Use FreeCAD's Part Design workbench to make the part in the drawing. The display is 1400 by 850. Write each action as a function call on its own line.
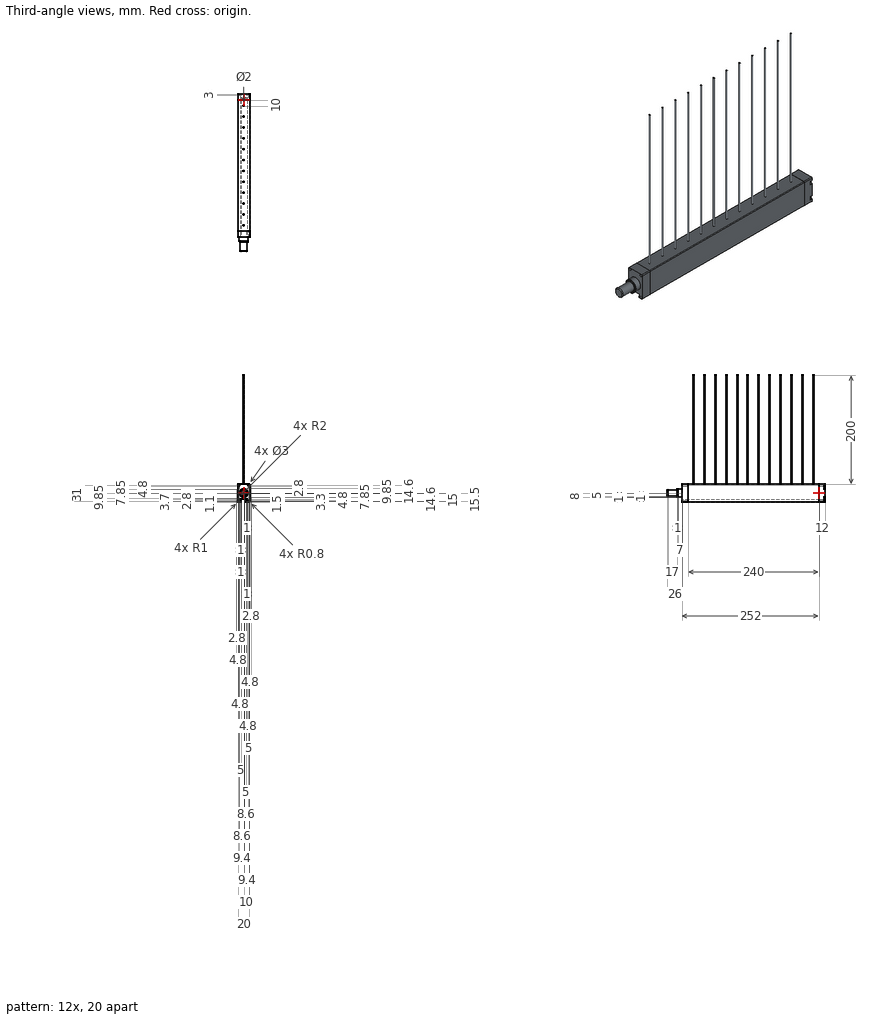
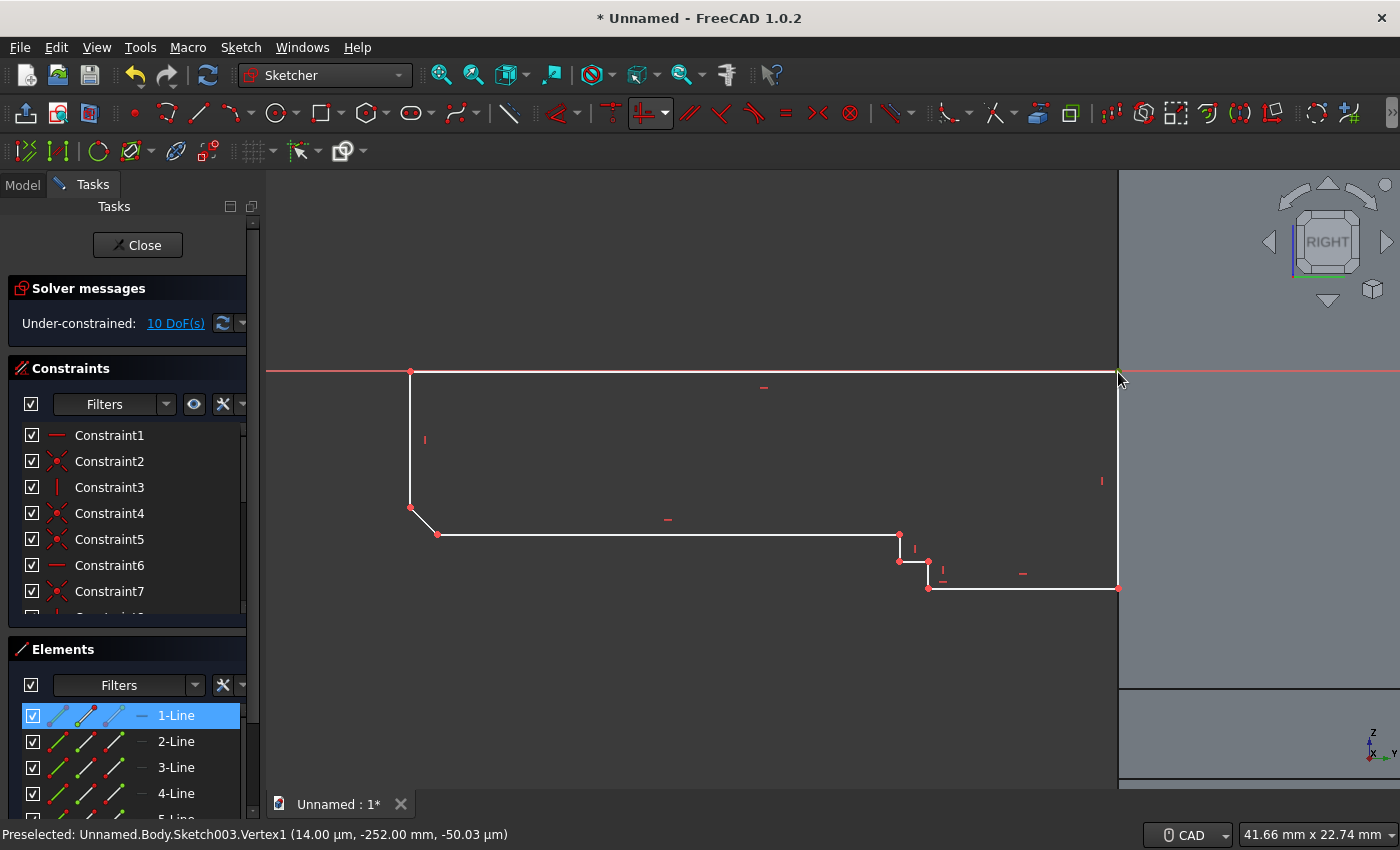
click(361, 371)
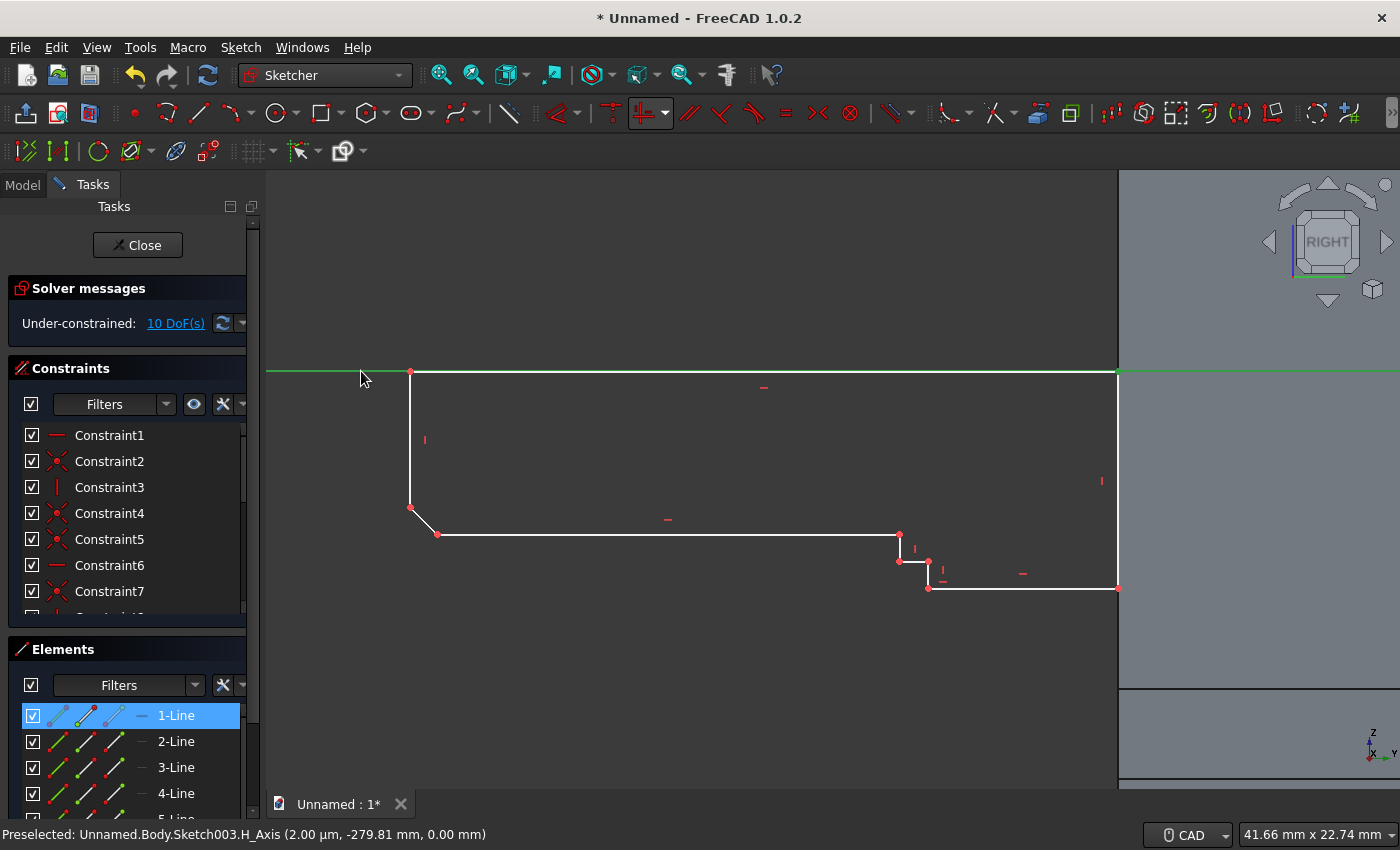
click(612, 114)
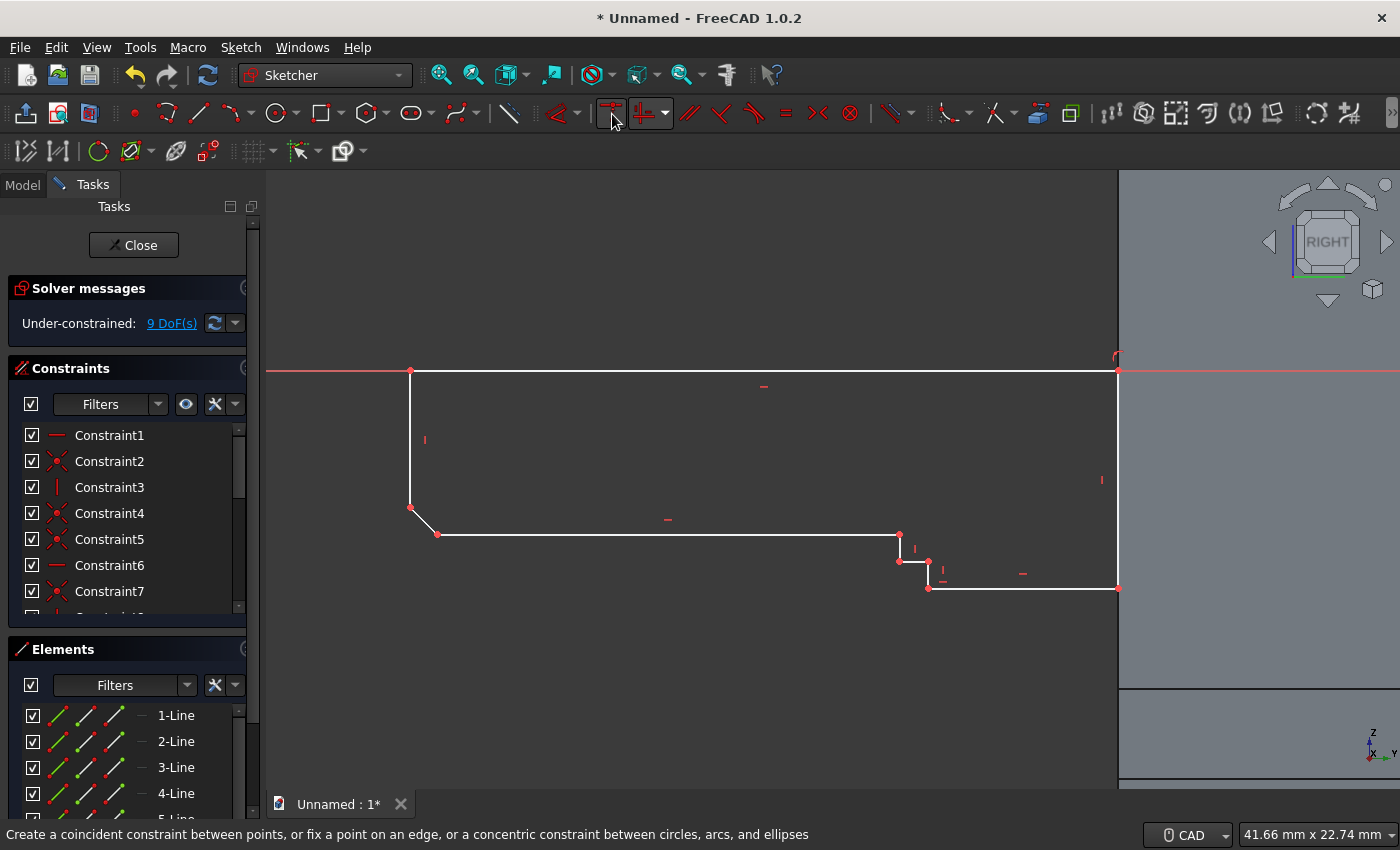
click(556, 114)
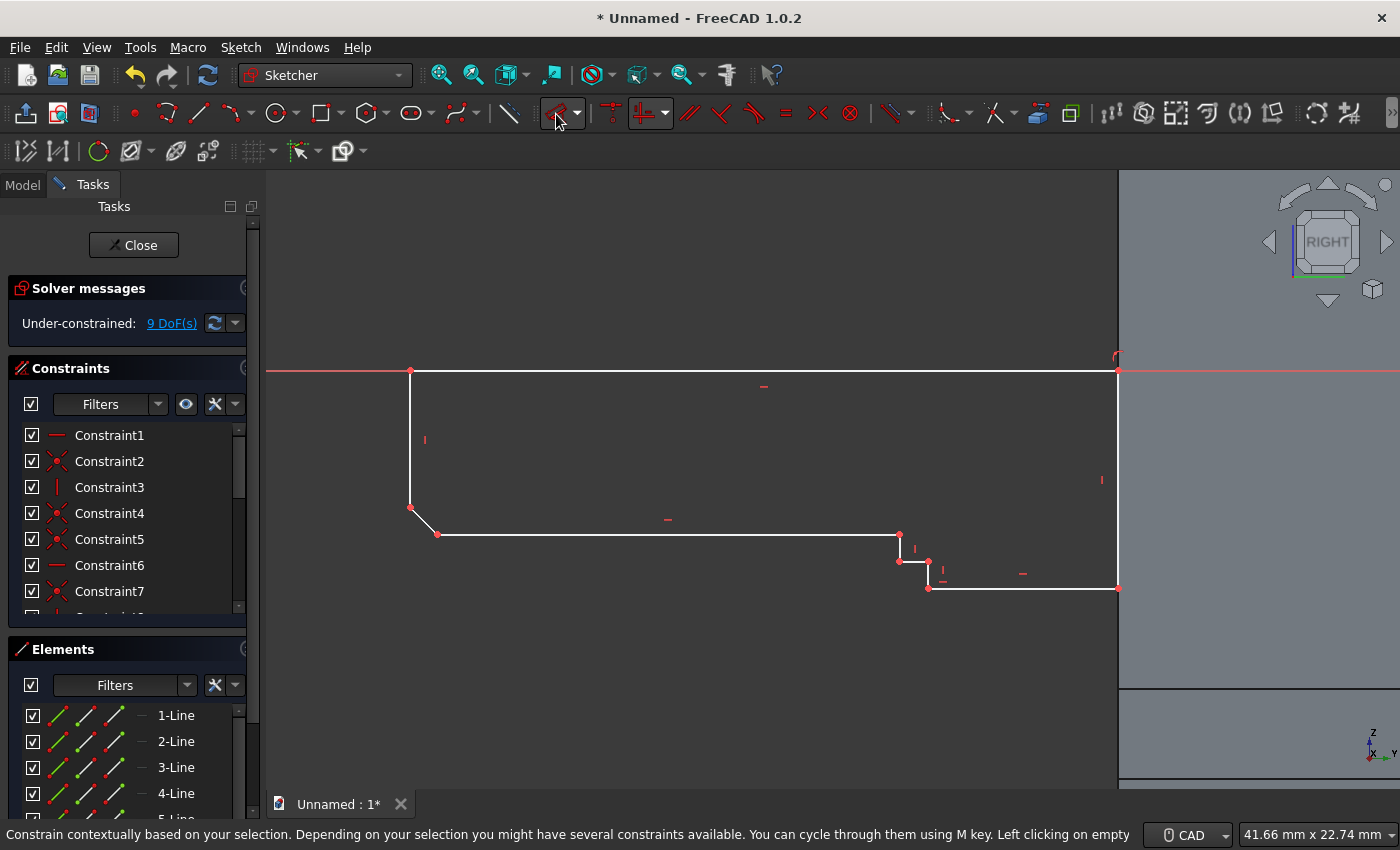
click(410, 412)
click(376, 439)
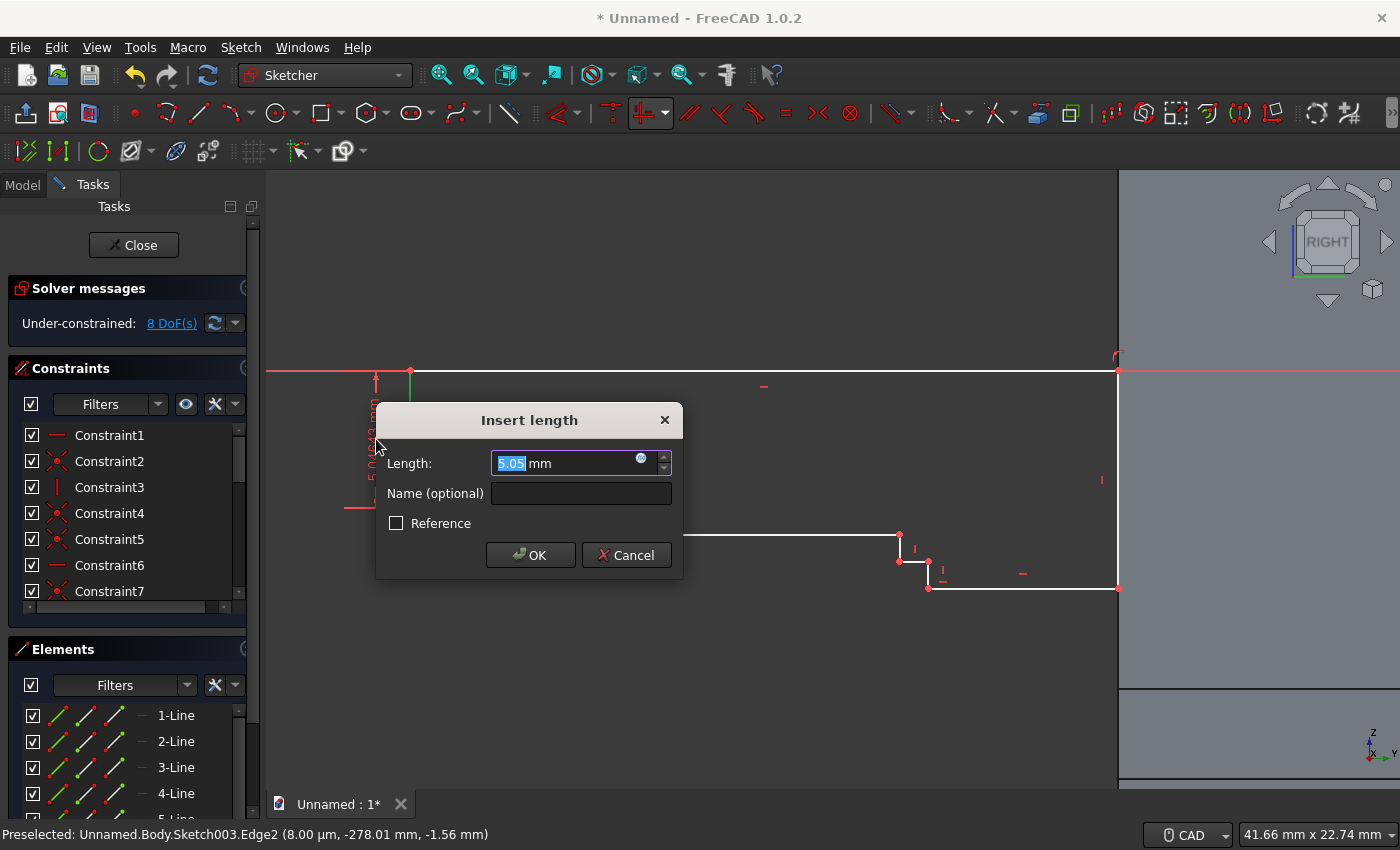
text(5)
key(Return)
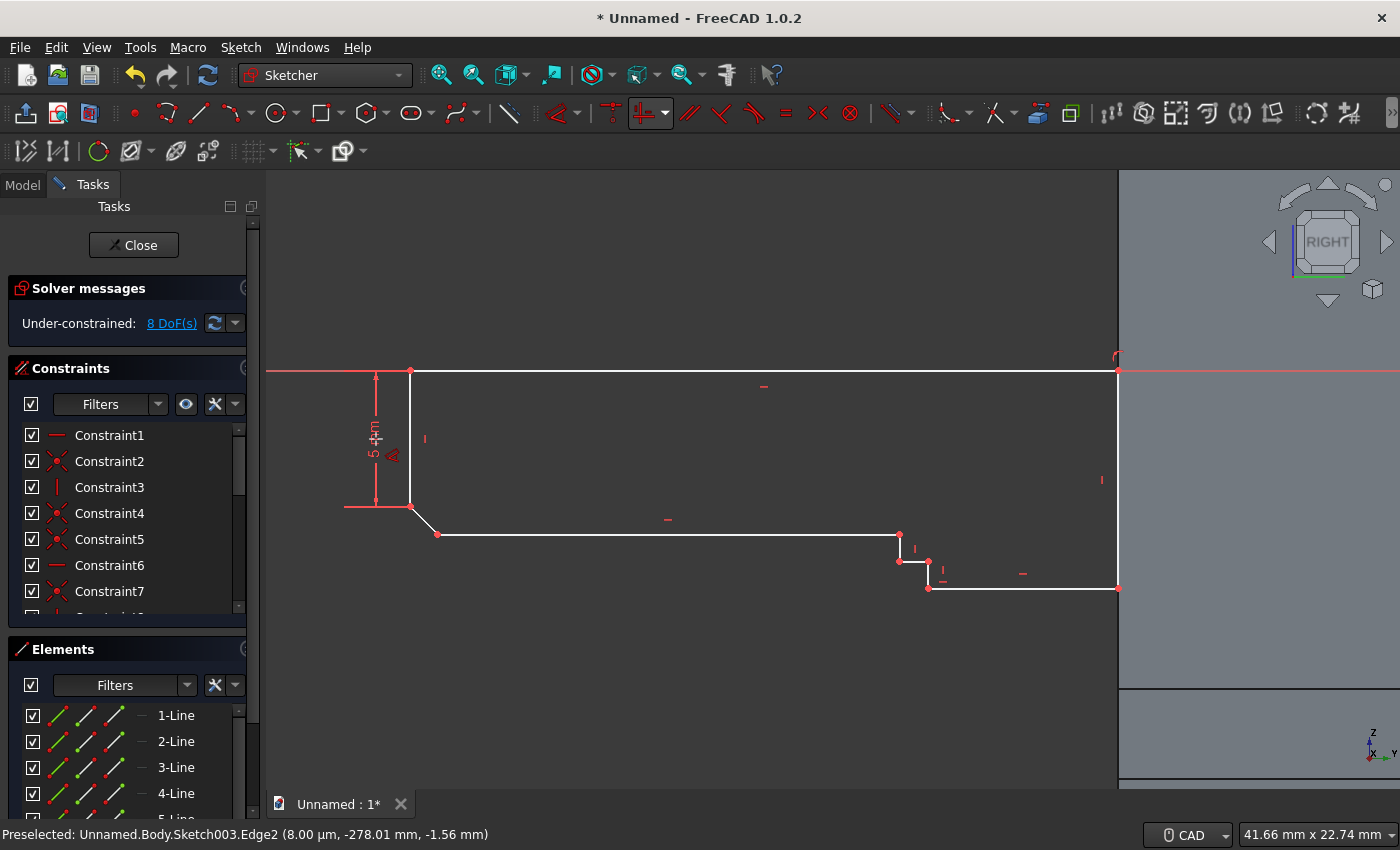
scroll(900, 546, up, 2)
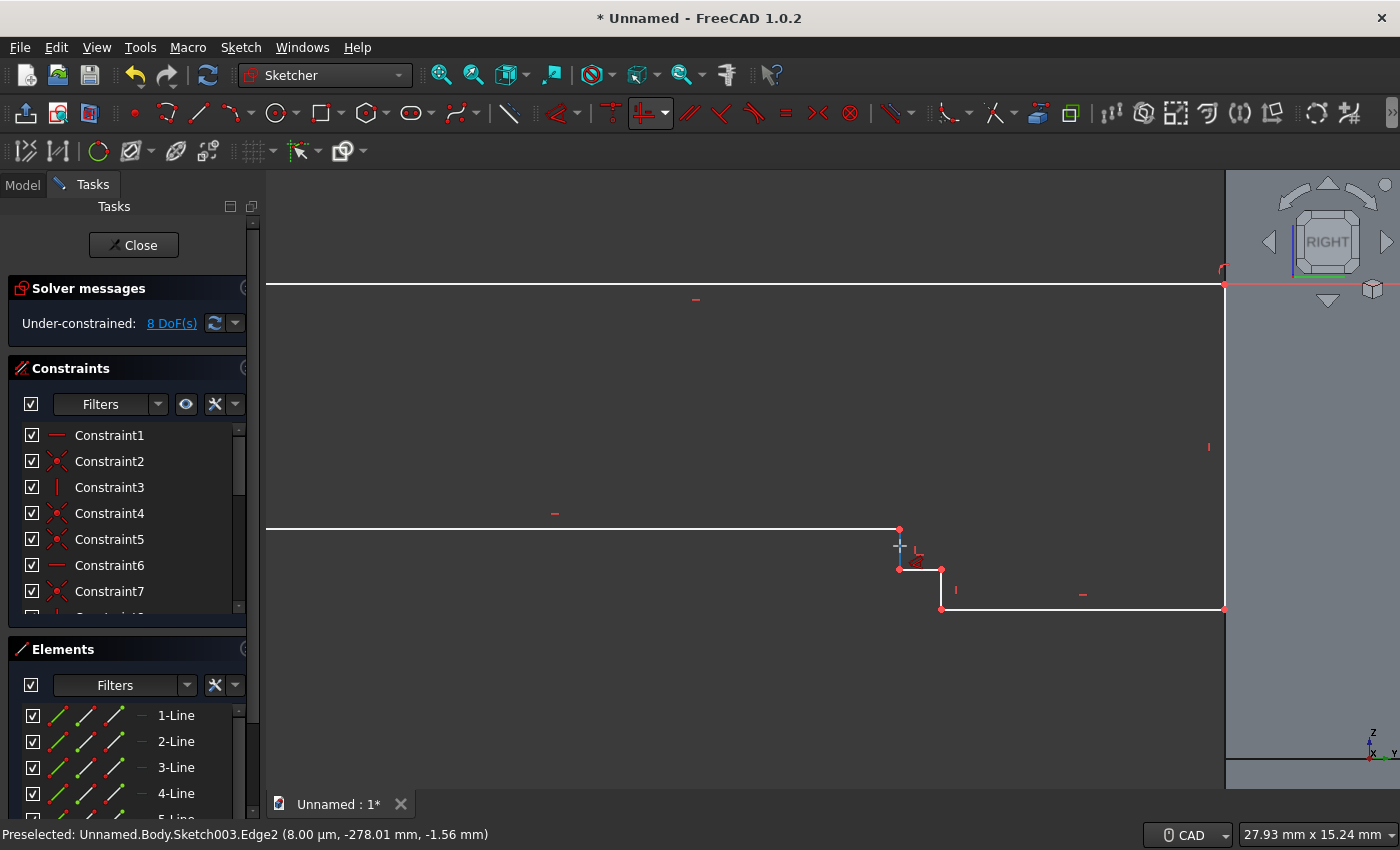
click(900, 545)
click(934, 549)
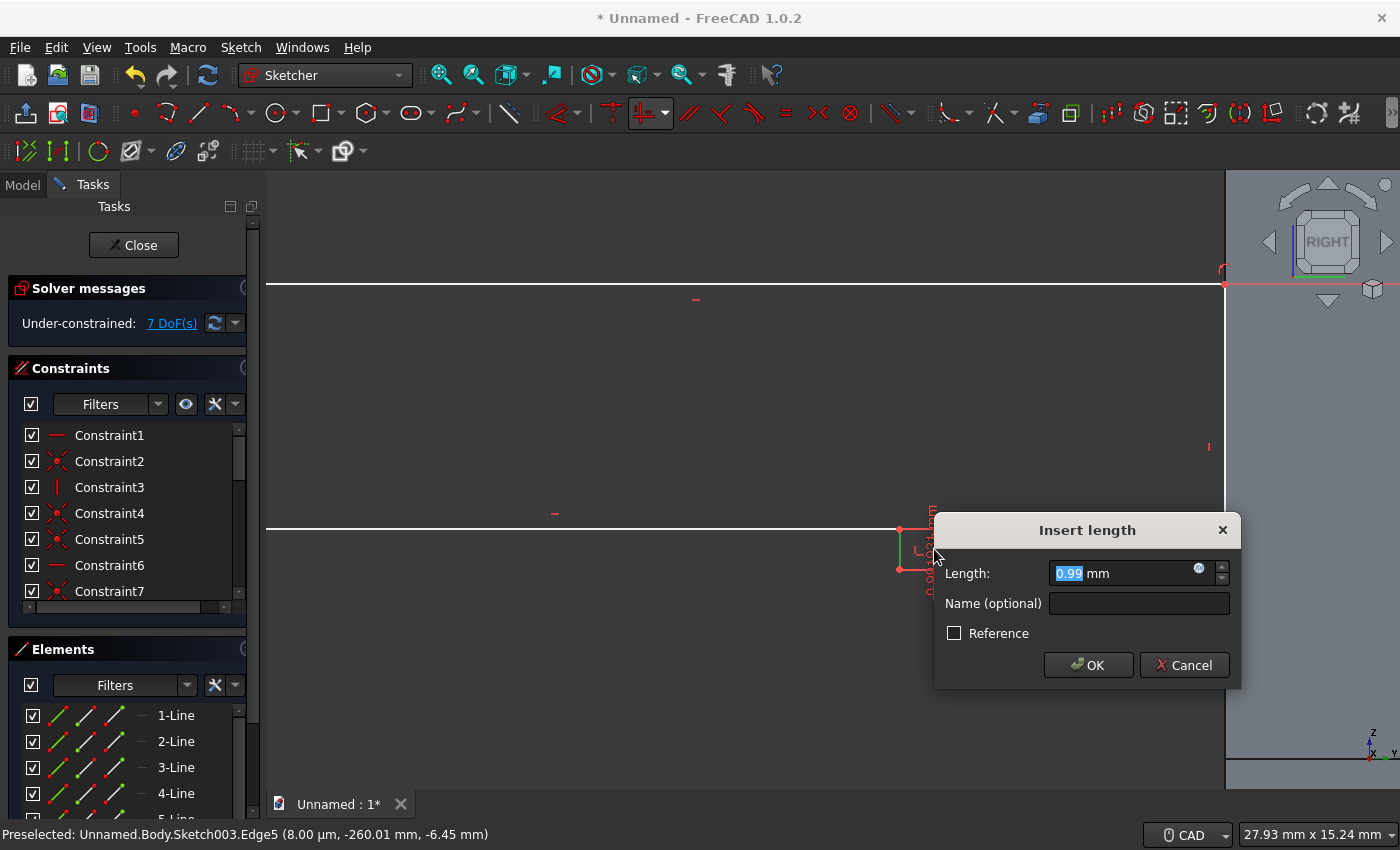
text(1)
key(Return)